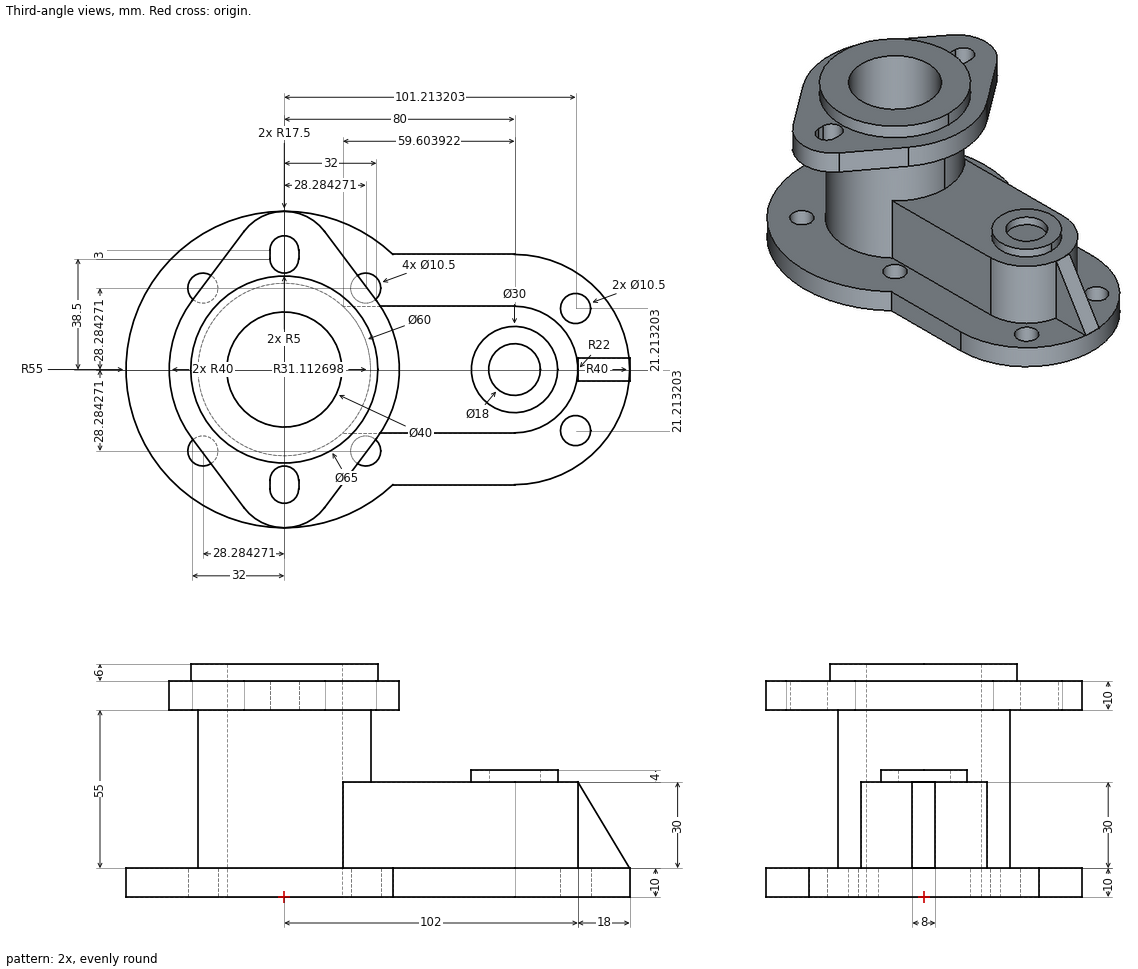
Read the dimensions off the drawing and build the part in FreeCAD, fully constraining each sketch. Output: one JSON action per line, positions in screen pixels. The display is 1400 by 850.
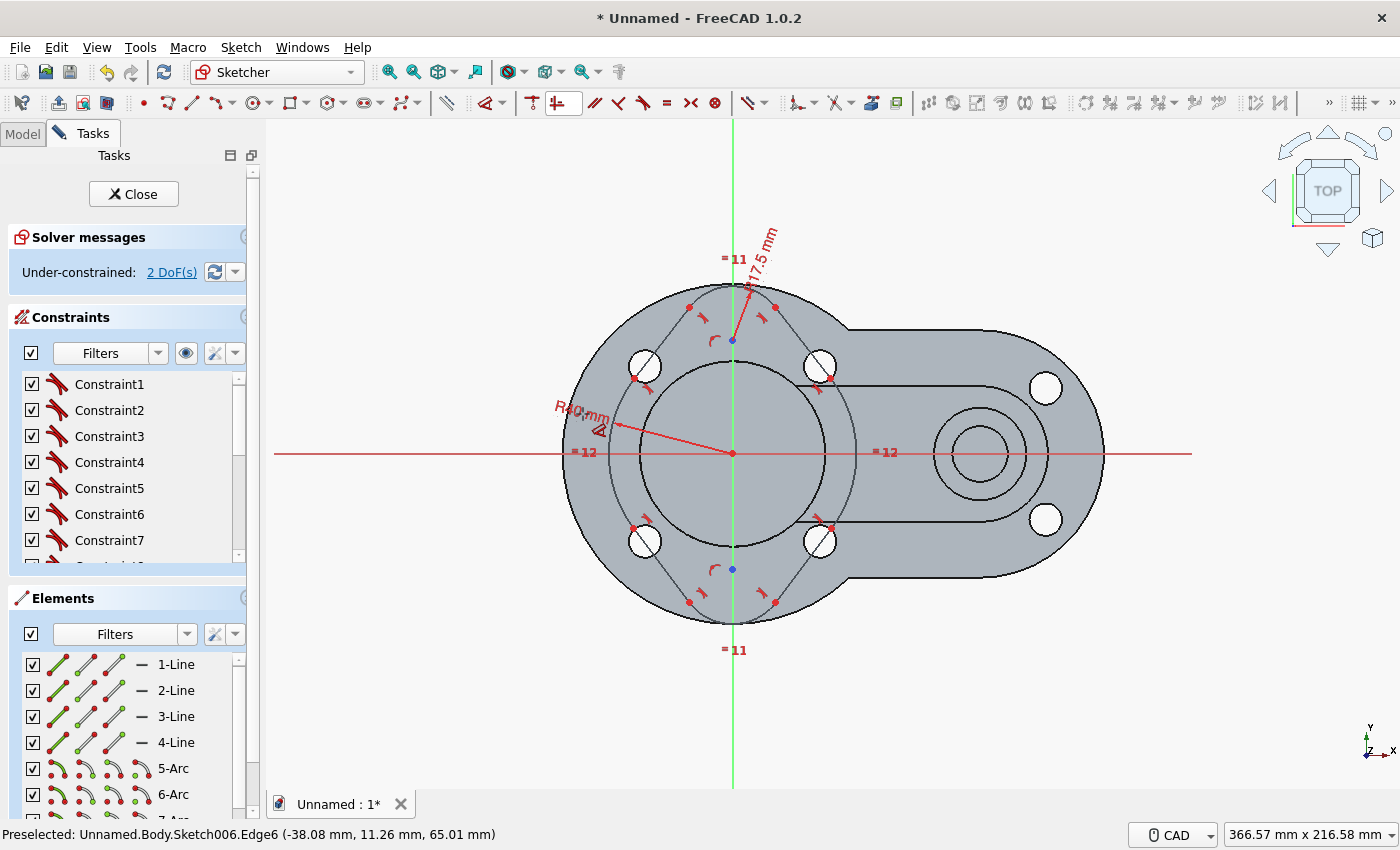
{"action": "left_click", "coordinate": [830, 378]}
{"action": "left_click", "coordinate": [782, 344]}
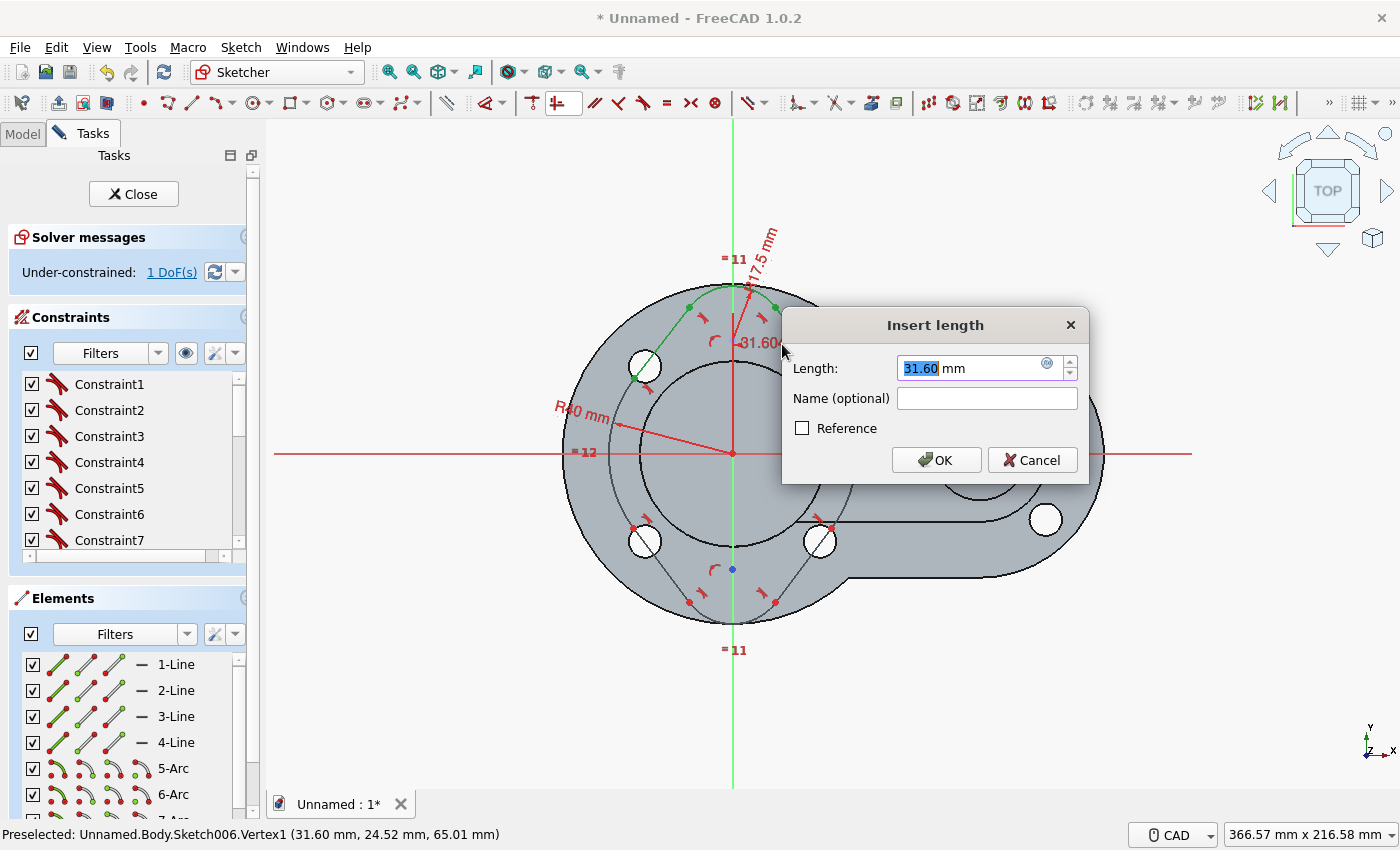
{"action": "type", "text": "32"}
{"action": "key", "text": "Return"}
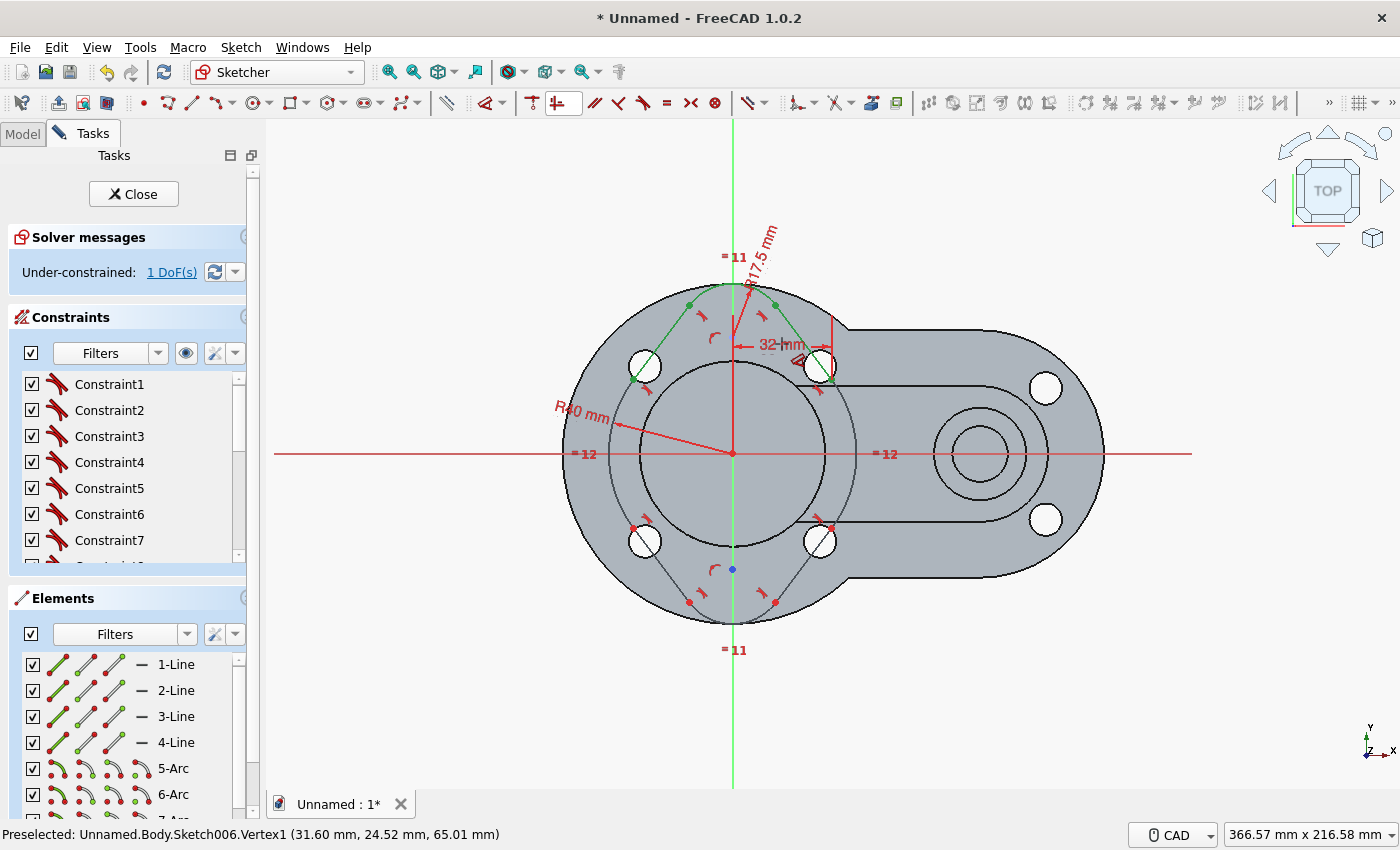
{"action": "left_click", "coordinate": [634, 528]}
{"action": "left_click", "coordinate": [683, 562]}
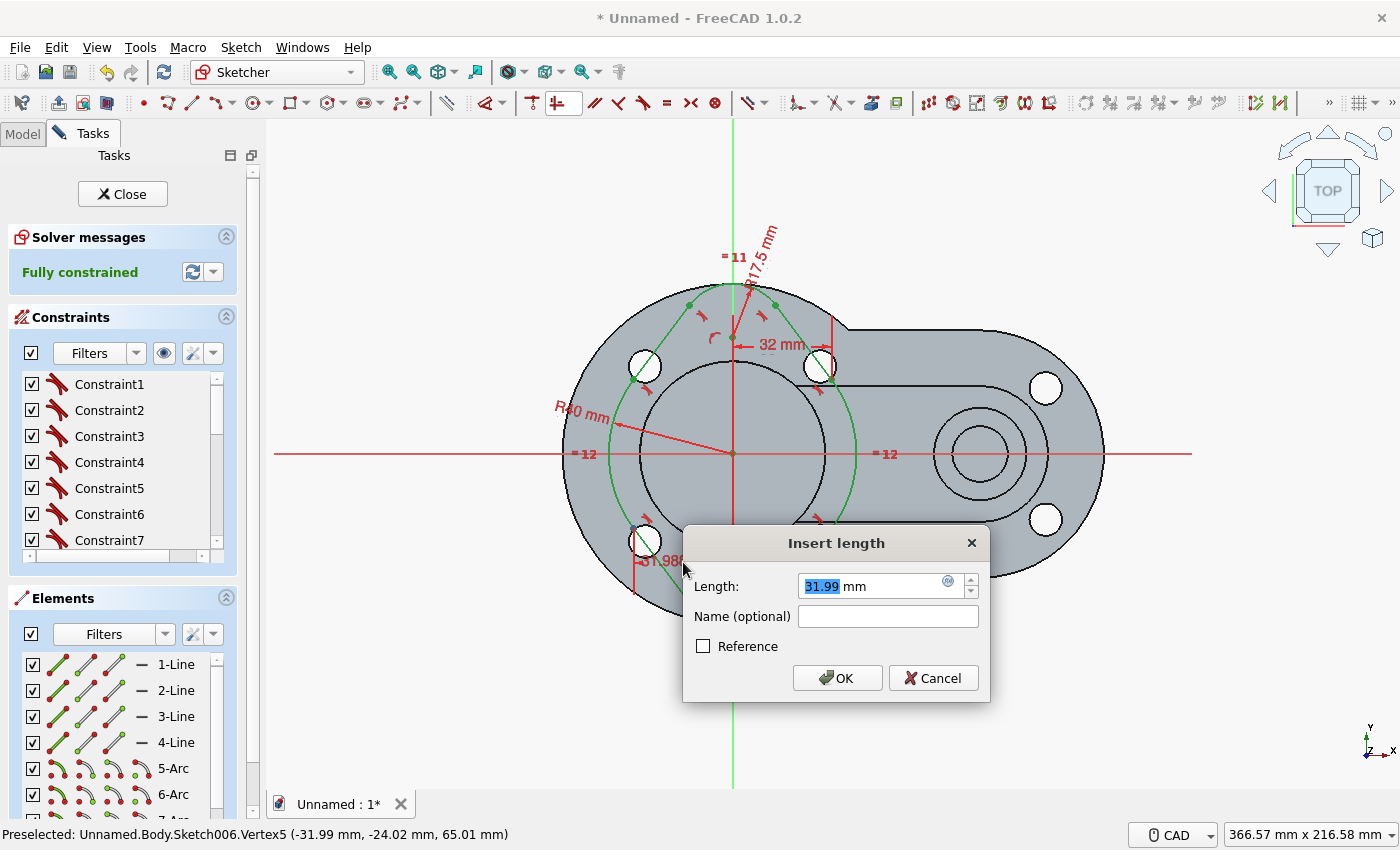
{"action": "type", "text": "32"}
{"action": "key", "text": "Return"}
{"action": "key", "text": "Escape"}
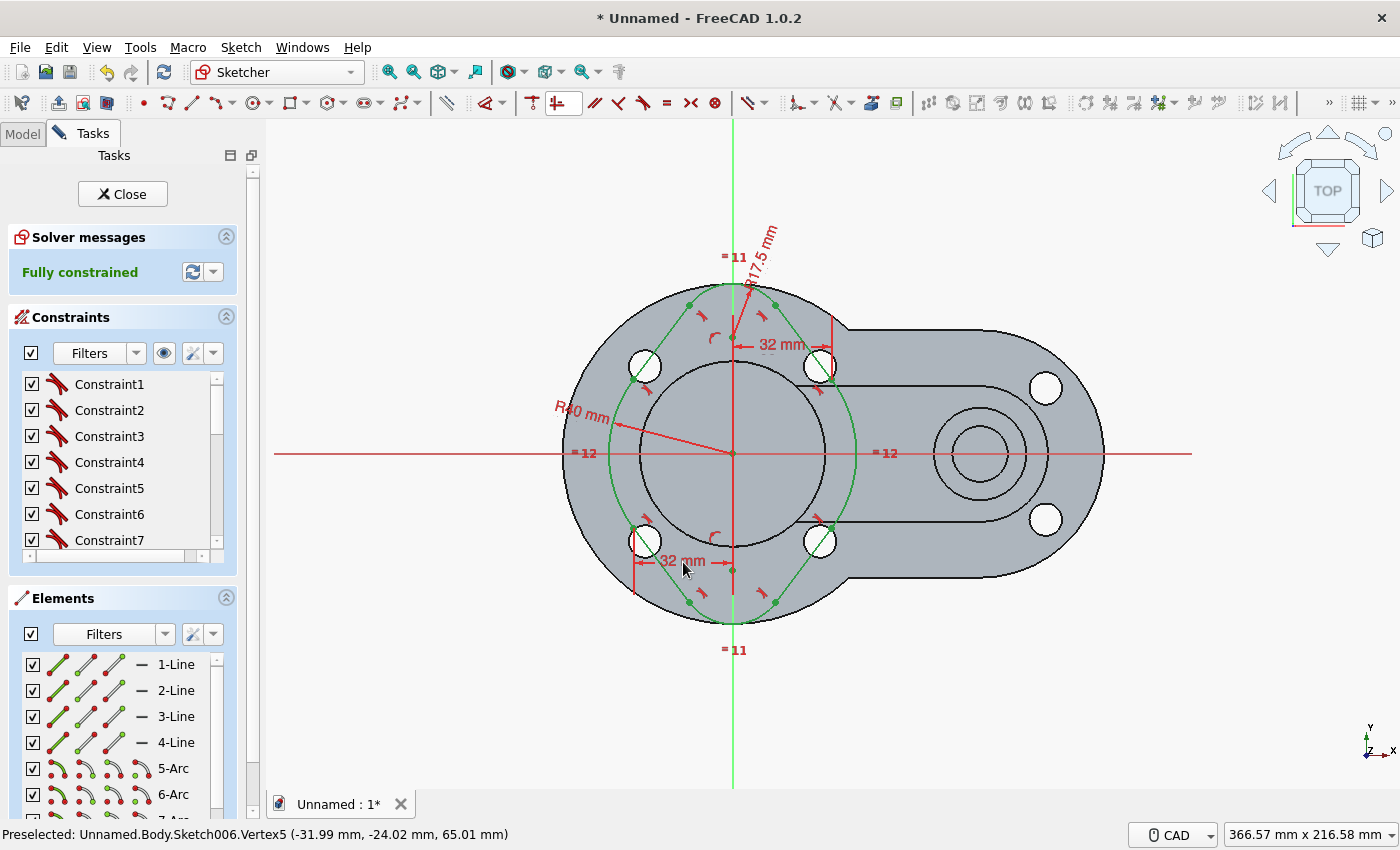
{"action": "left_click", "coordinate": [123, 194]}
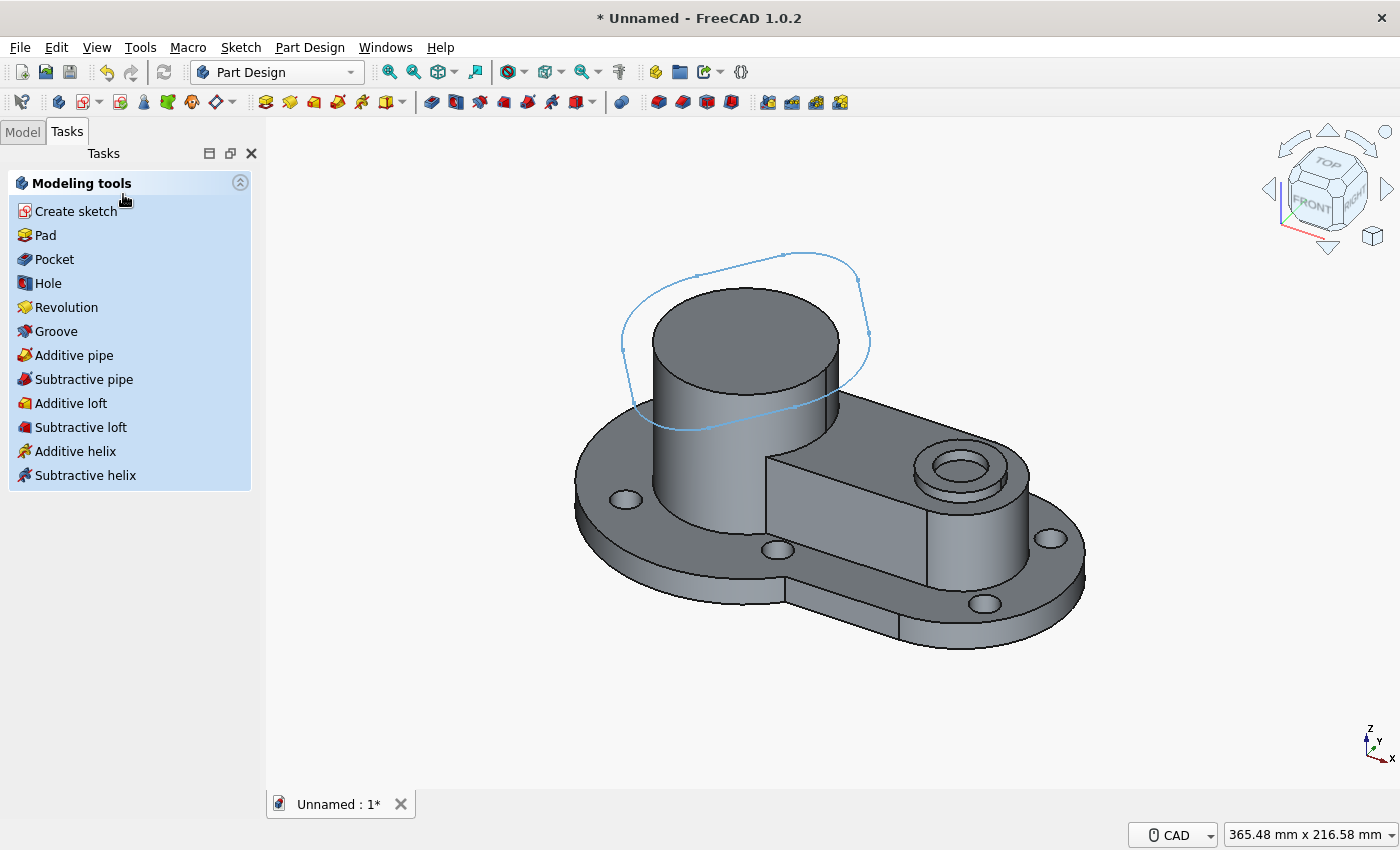
{"action": "left_click", "coordinate": [266, 102]}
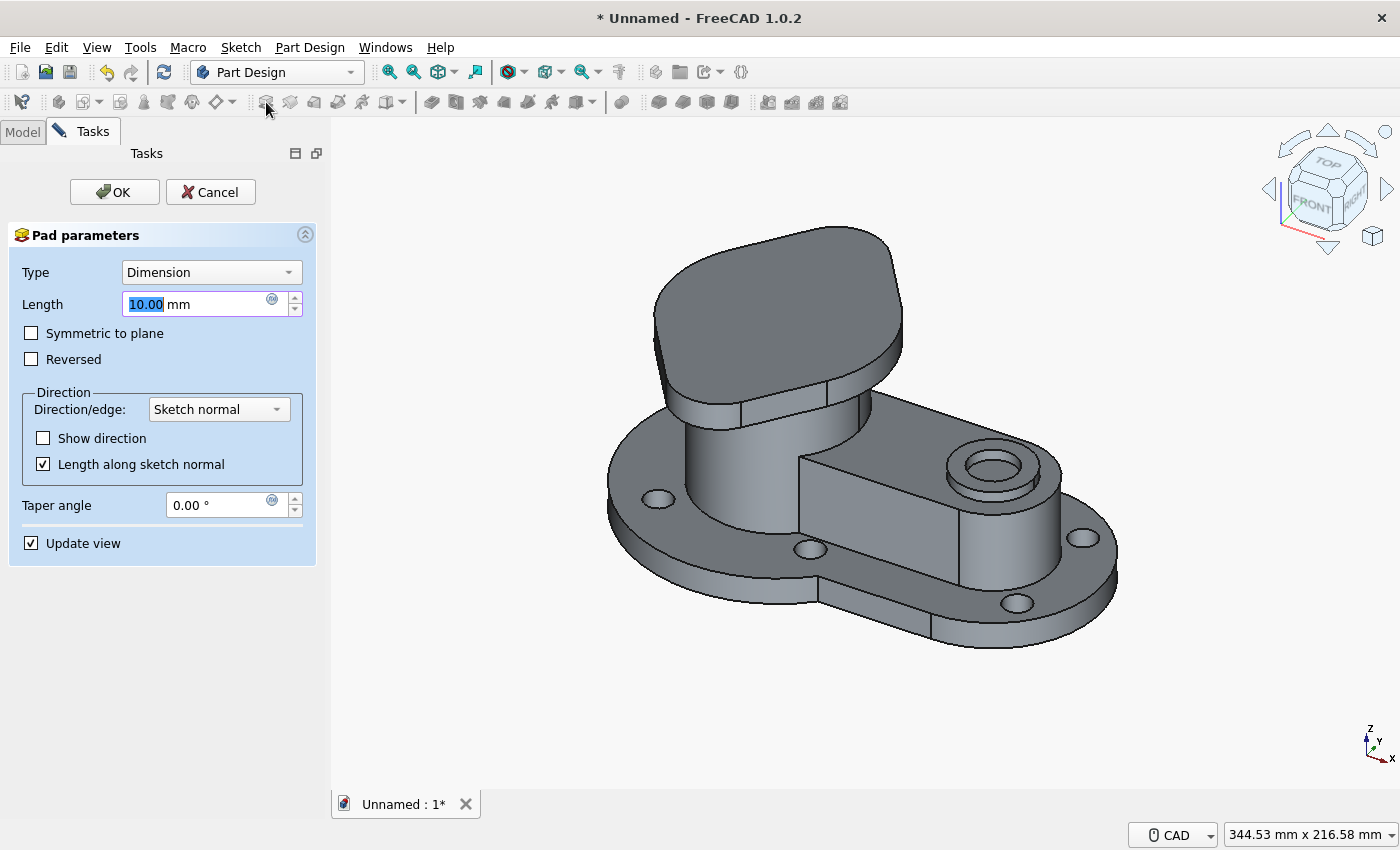
{"action": "type", "text": "10"}
{"action": "key", "text": "Tab"}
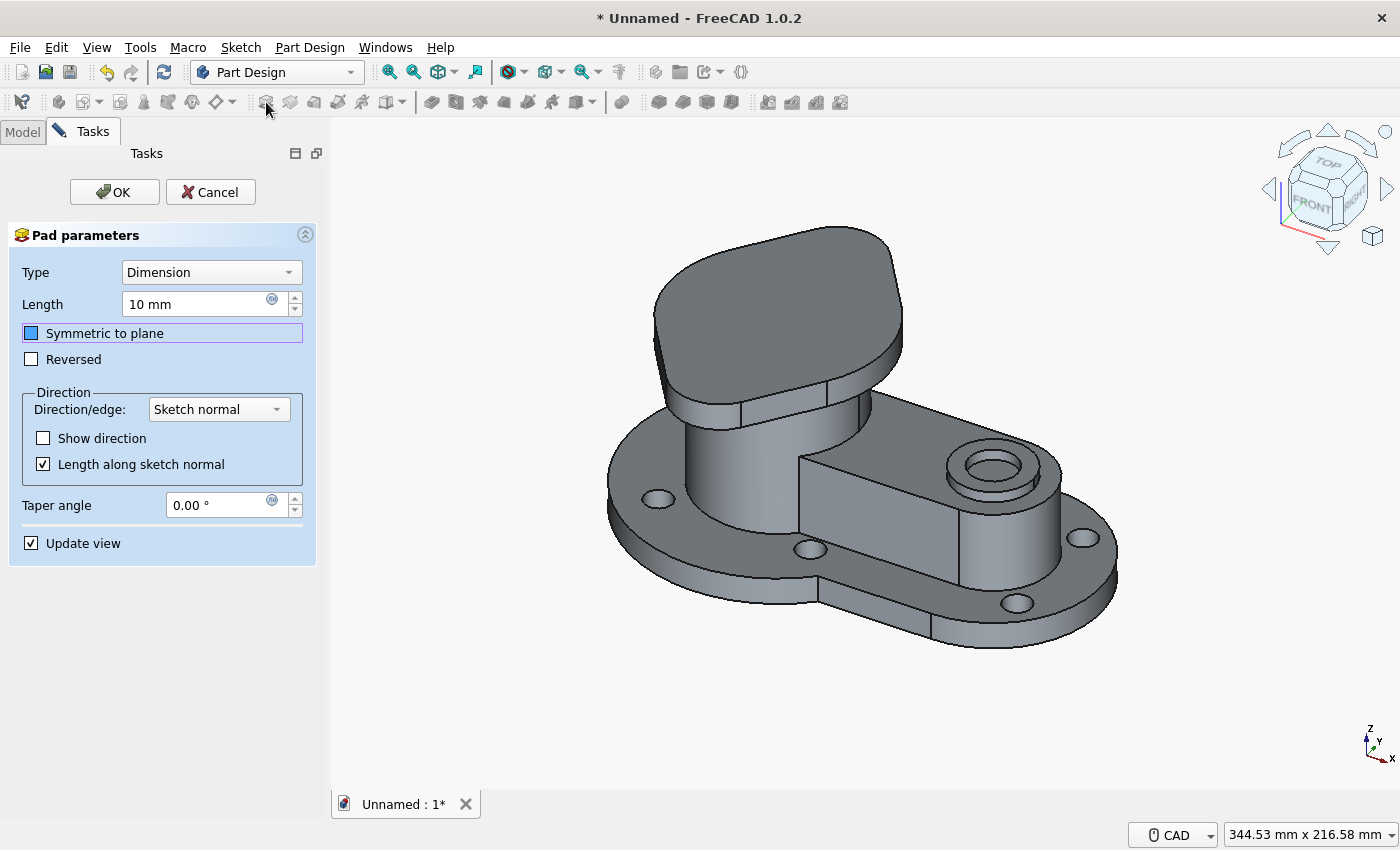
{"action": "left_click", "coordinate": [115, 192]}